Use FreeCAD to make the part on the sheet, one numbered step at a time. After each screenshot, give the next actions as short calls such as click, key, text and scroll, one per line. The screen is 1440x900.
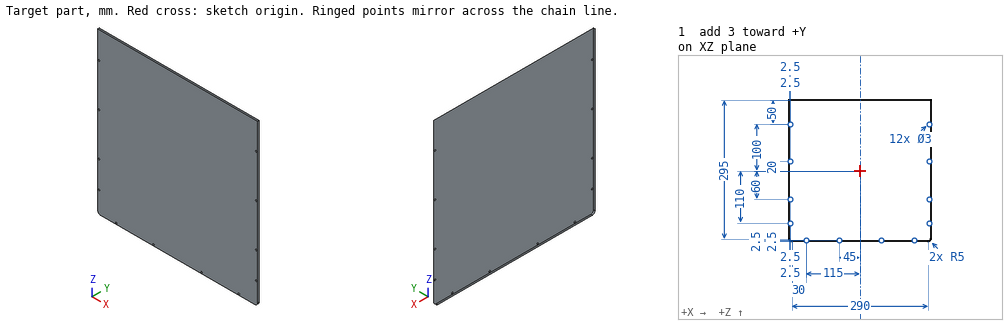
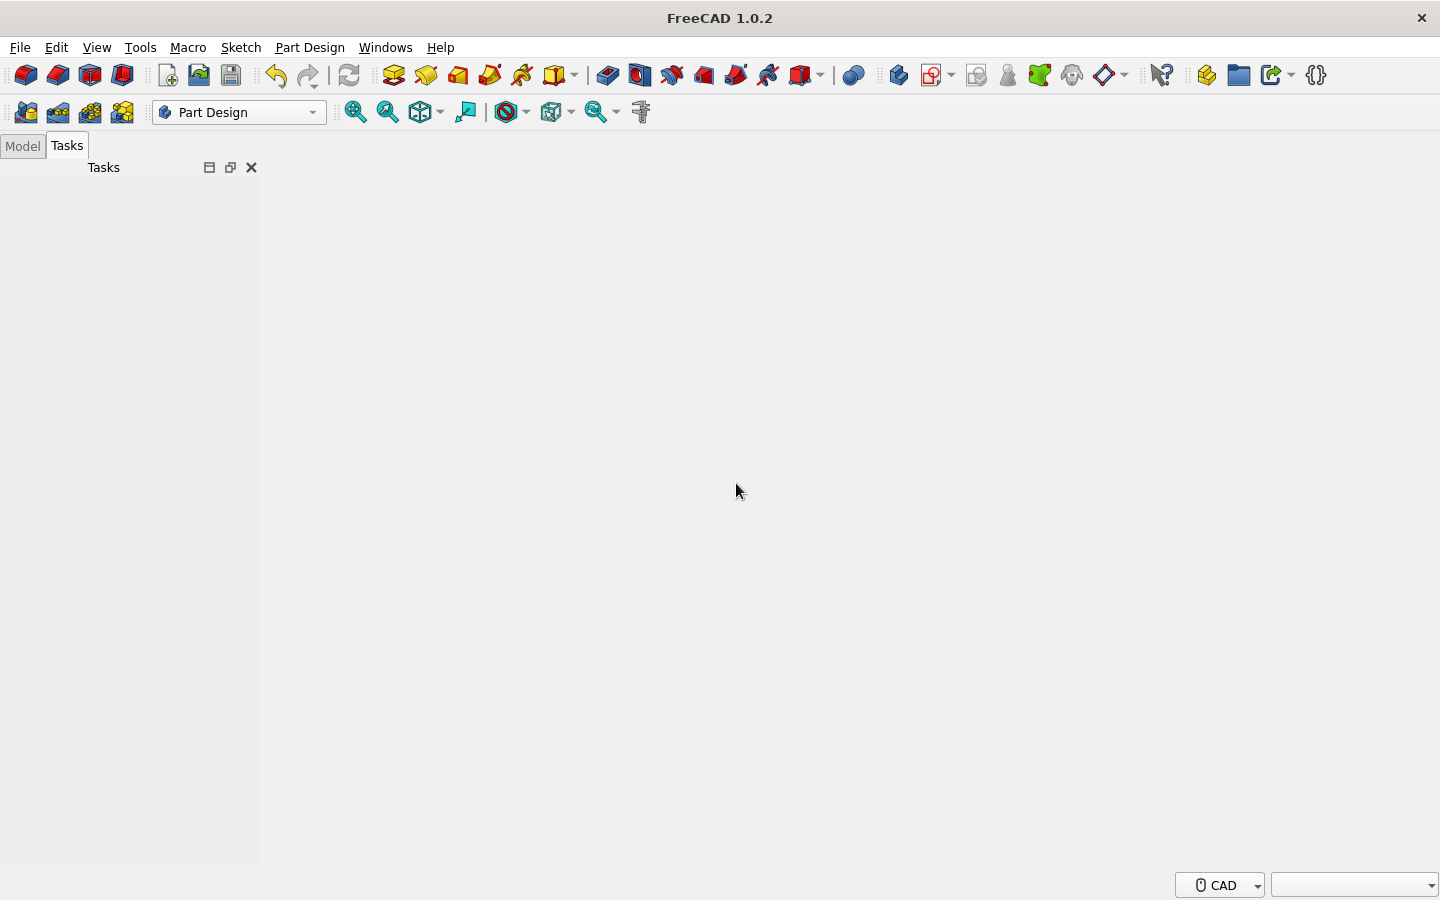
click(168, 76)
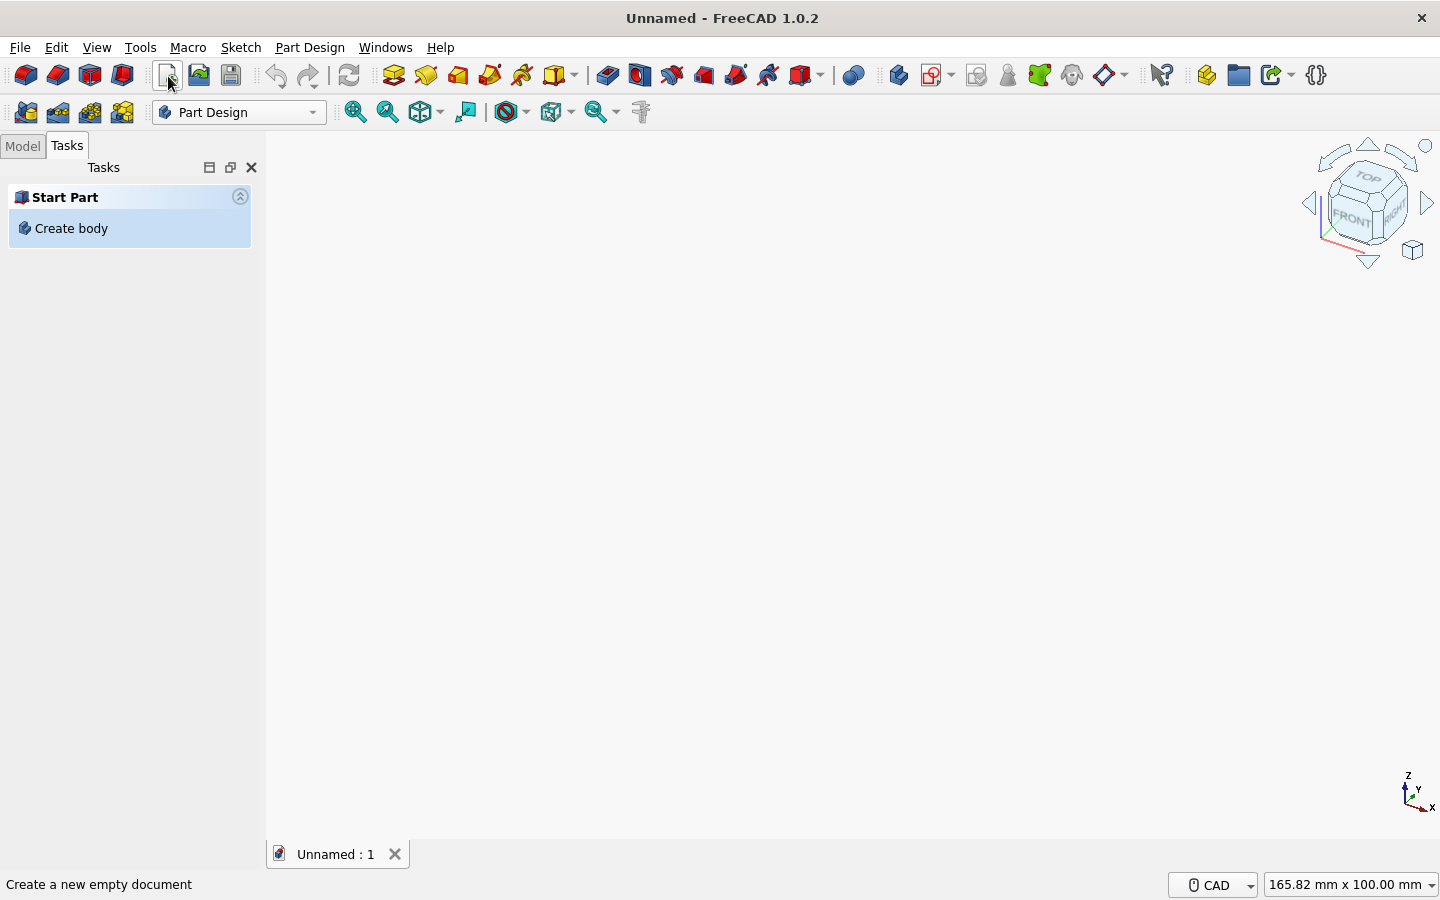
click(932, 76)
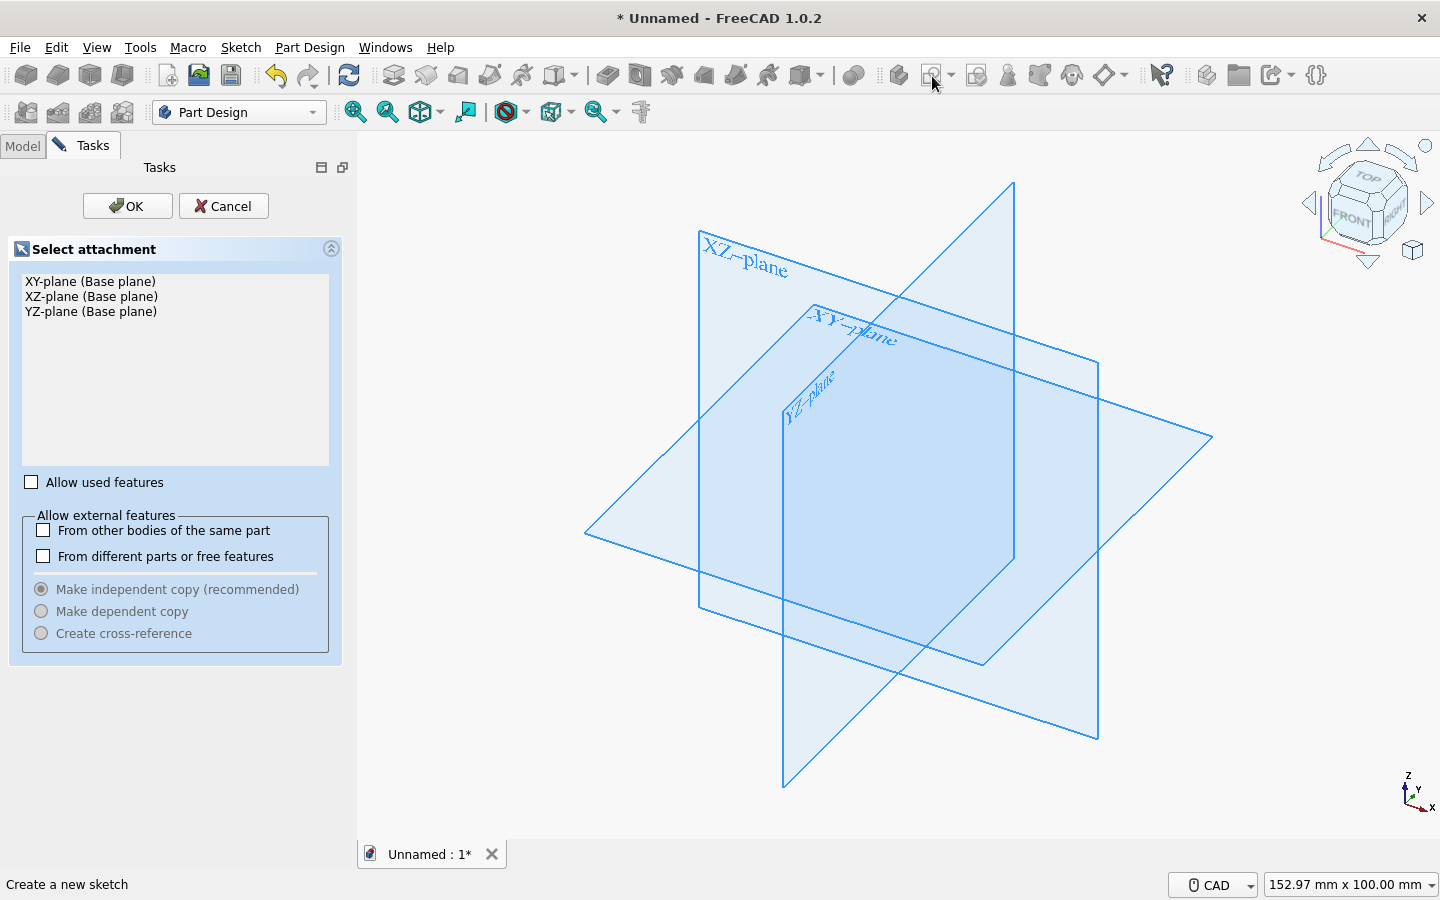
click(82, 296)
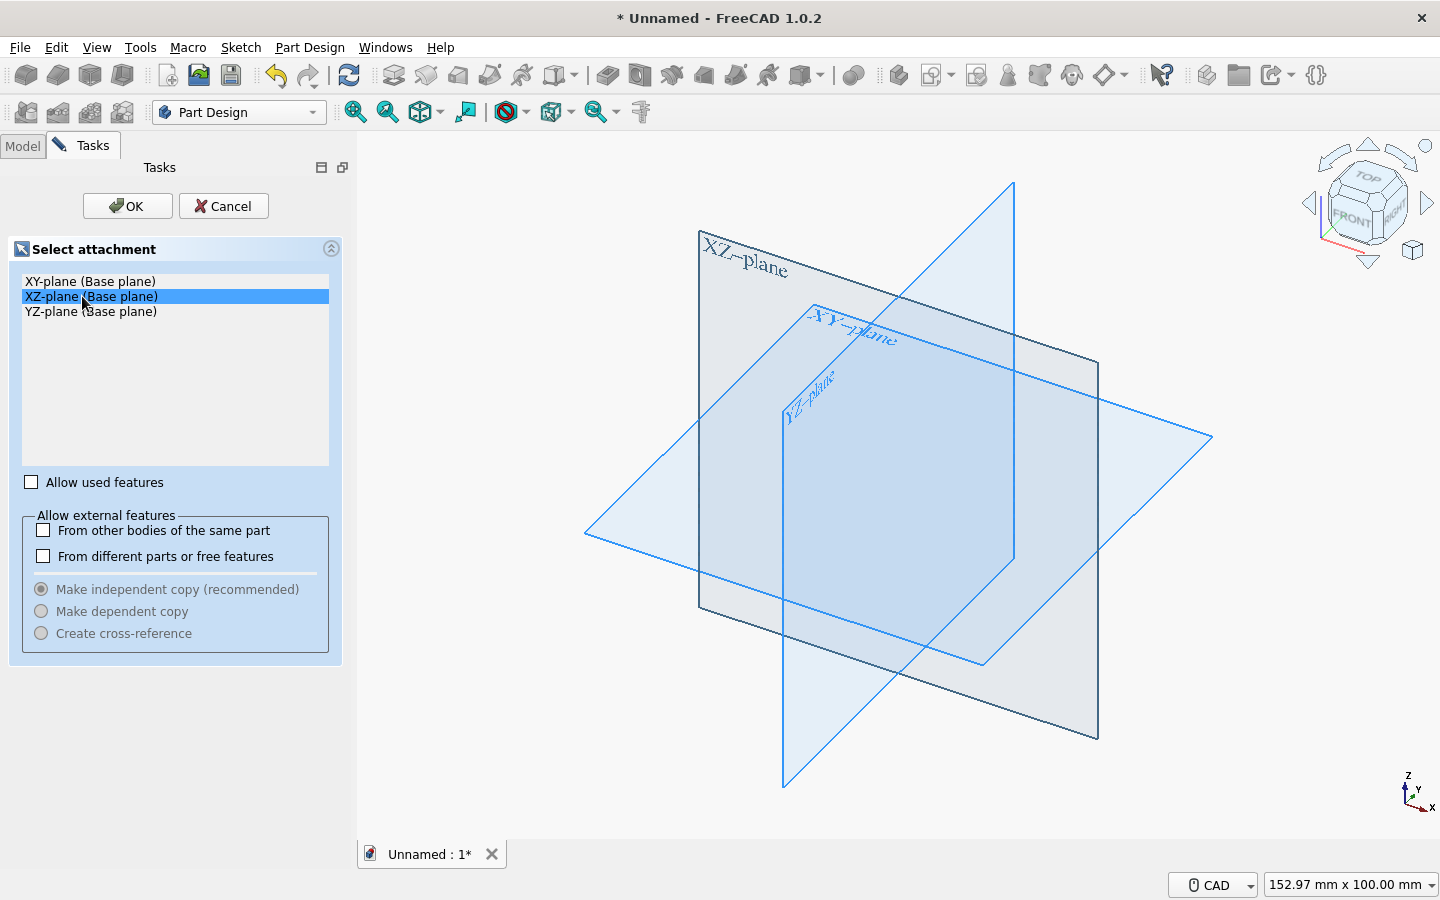
click(128, 206)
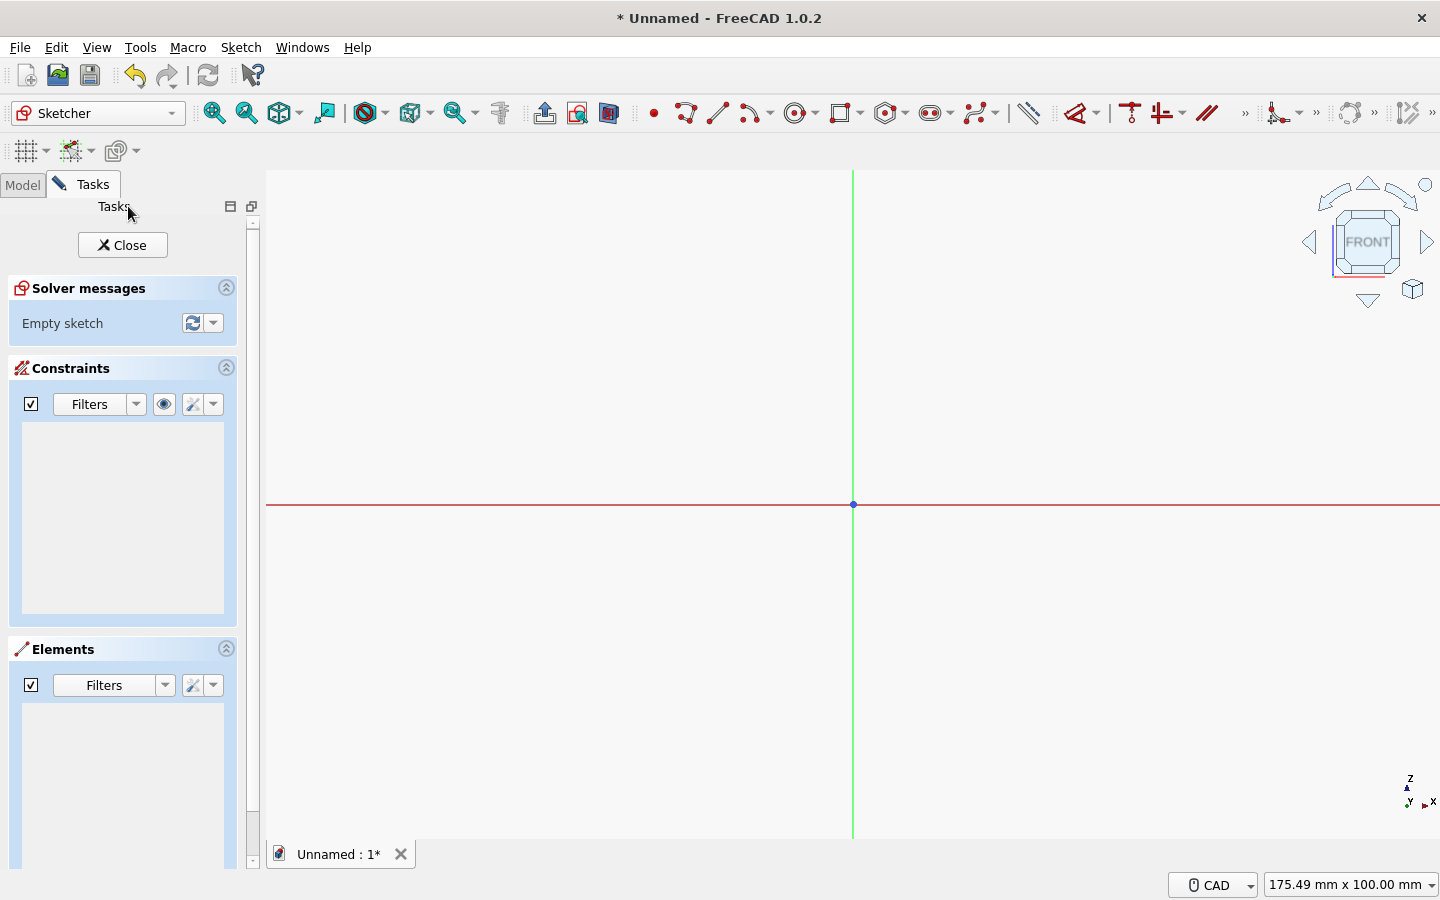
scroll(767, 504, down, 8)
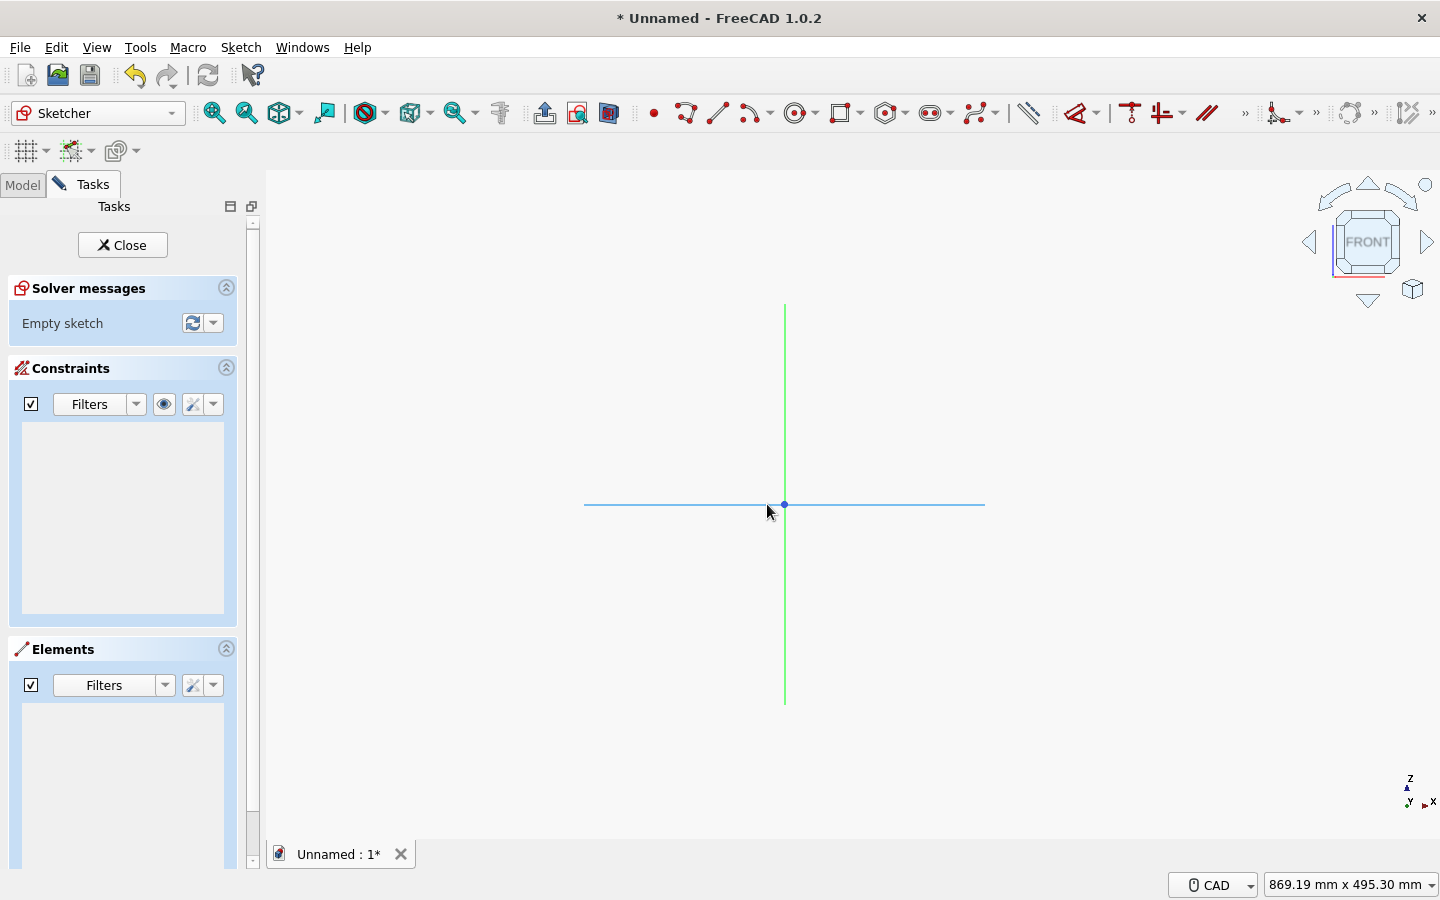
click(718, 114)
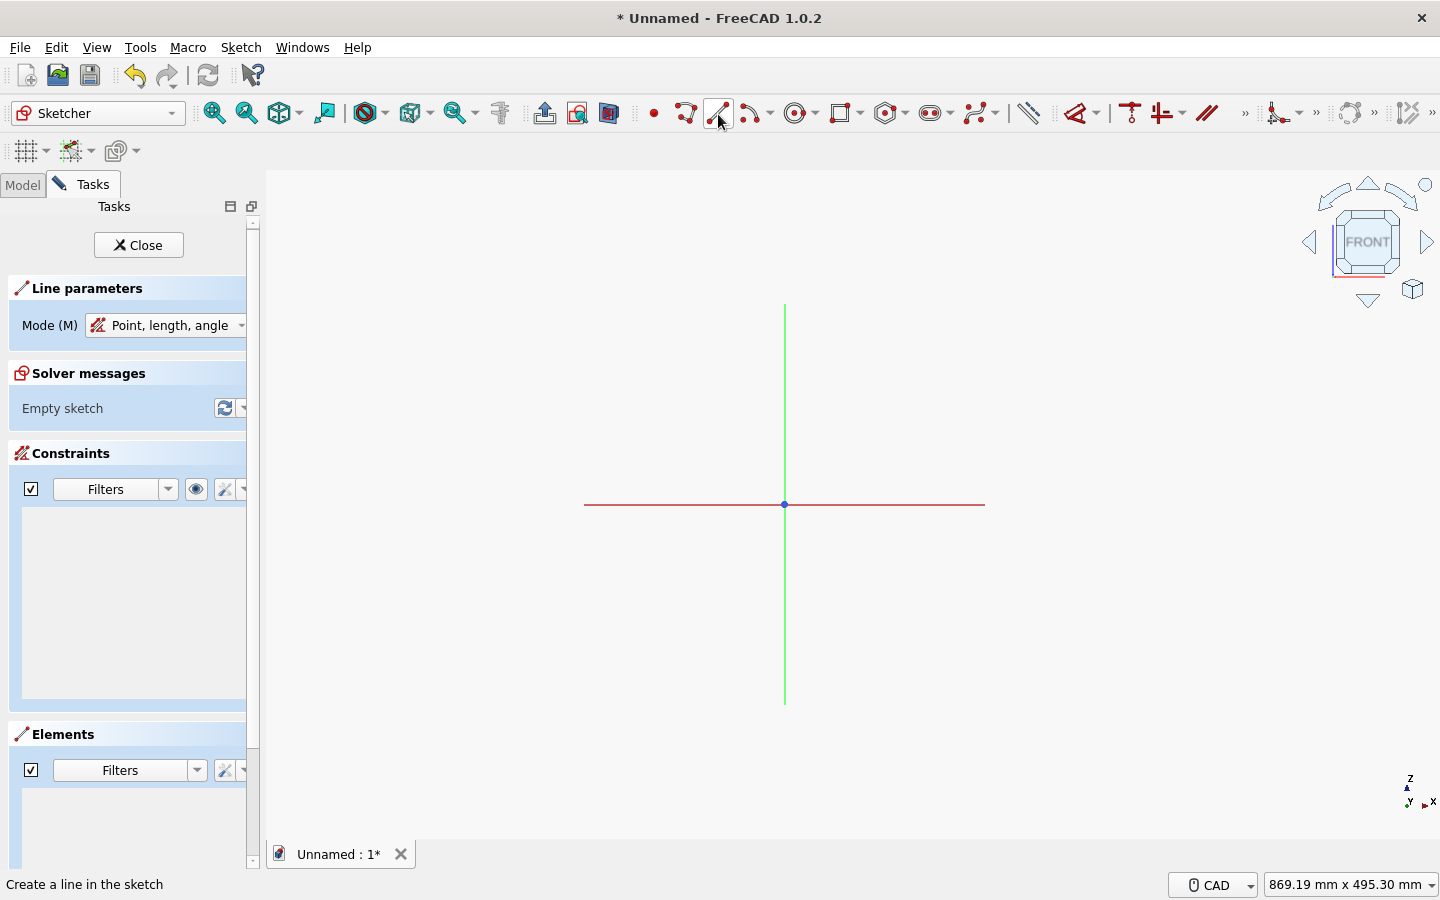
click(981, 707)
click(589, 707)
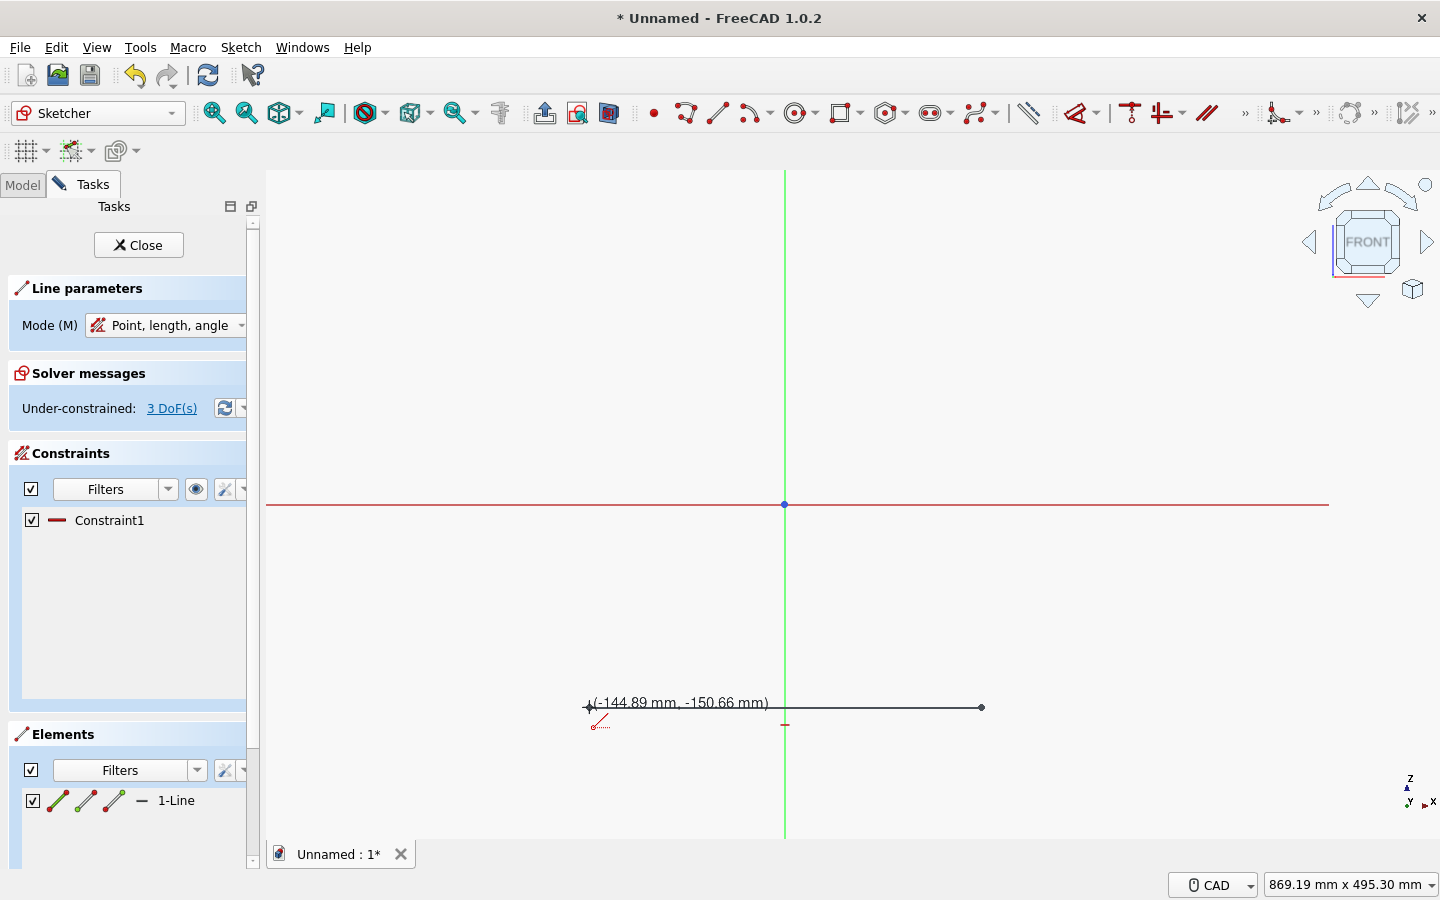
click(686, 114)